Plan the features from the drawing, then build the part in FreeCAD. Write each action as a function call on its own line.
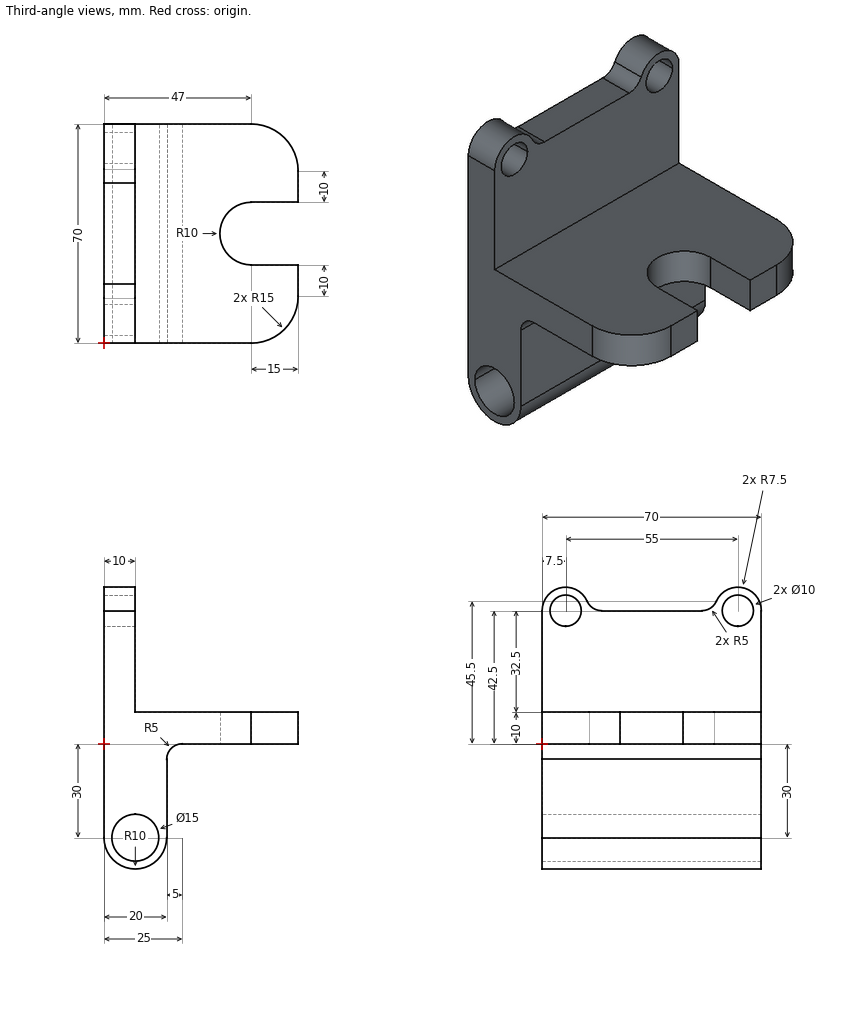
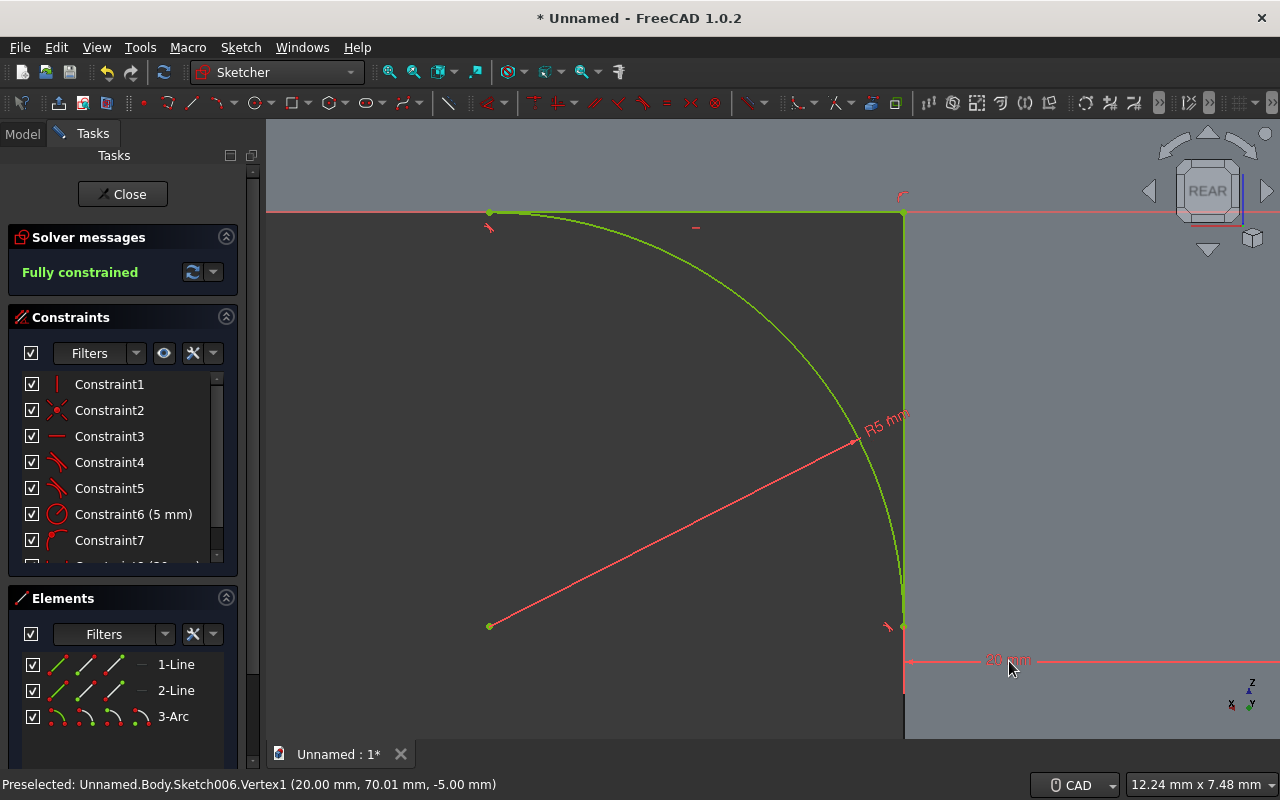
click(123, 194)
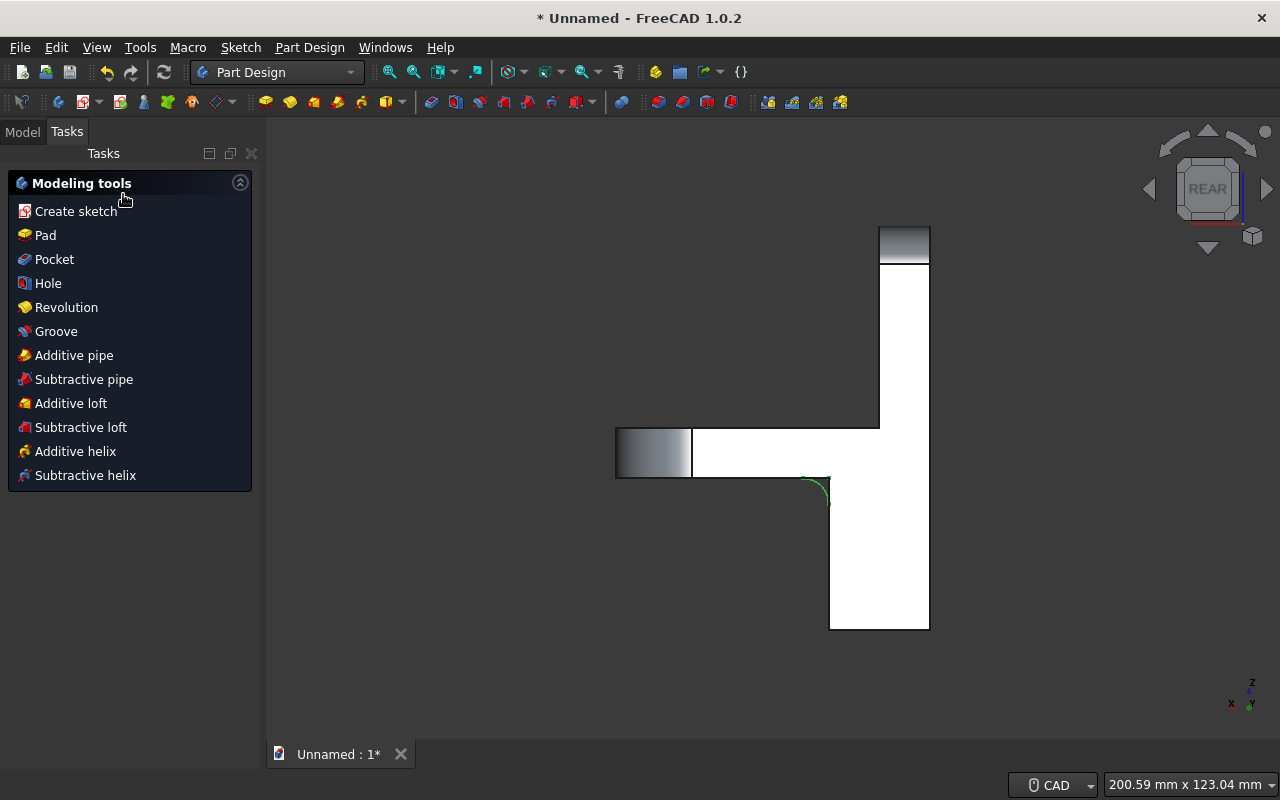
click(266, 102)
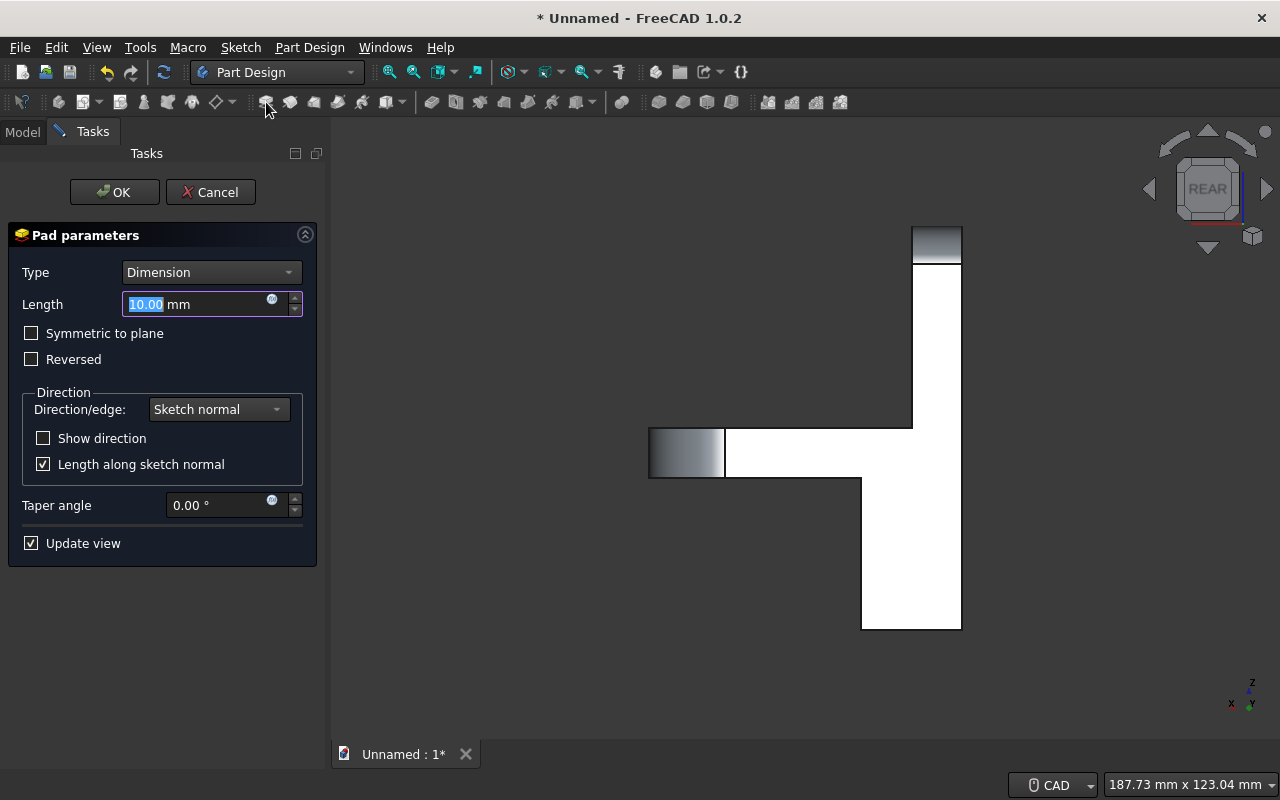
text(70)
key(Tab)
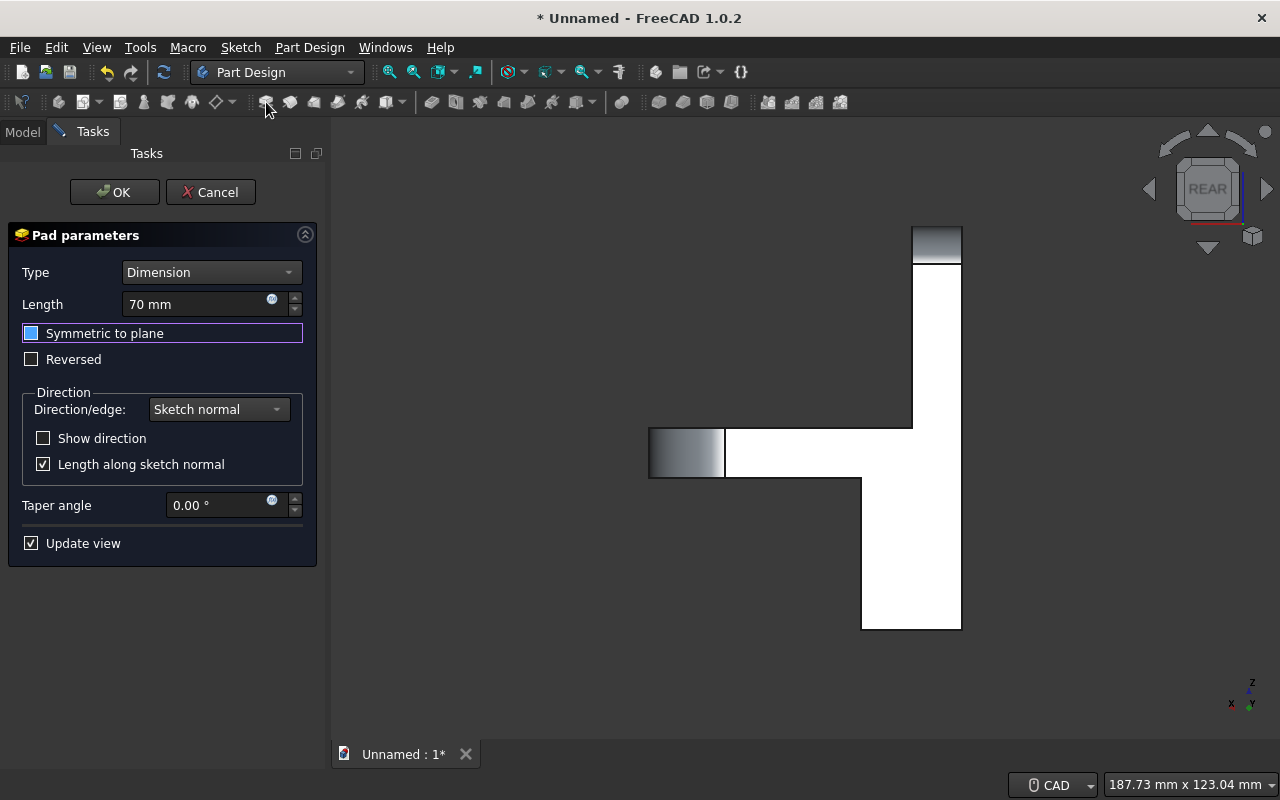
click(30, 359)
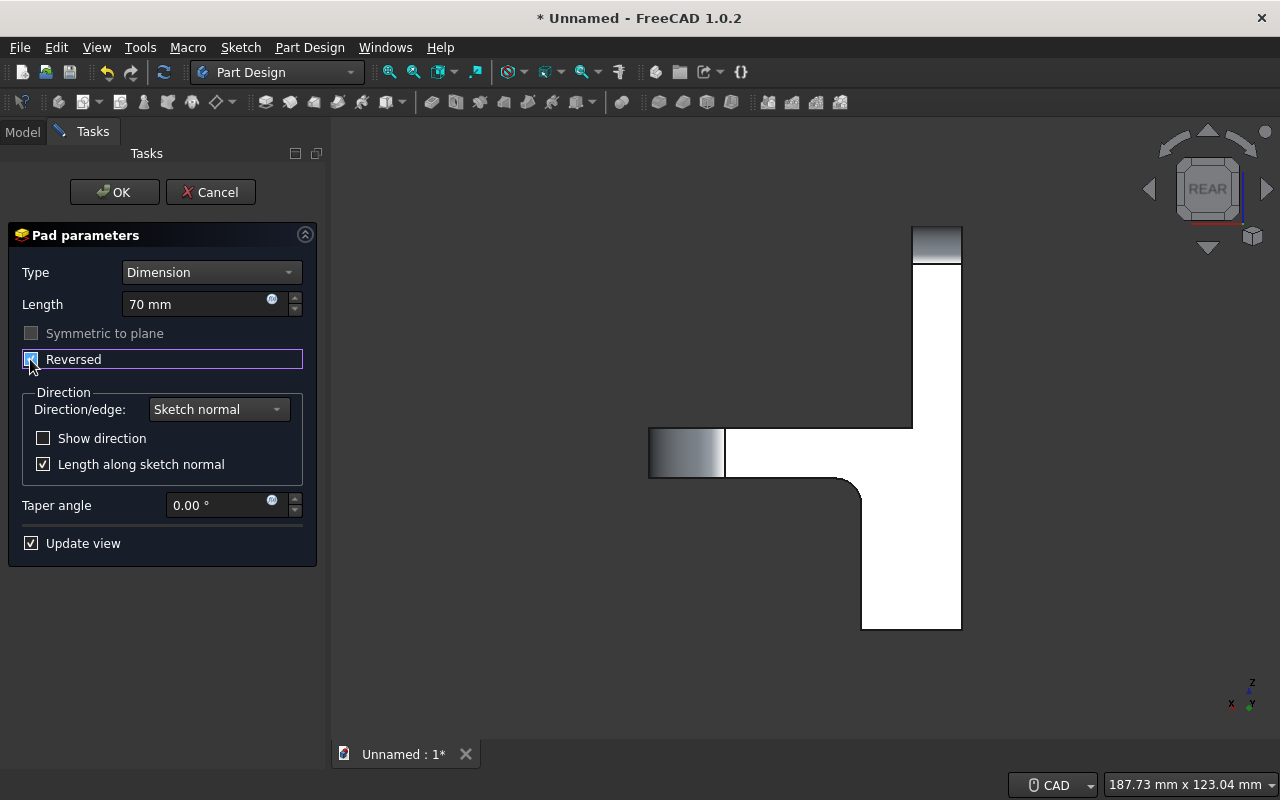
click(115, 192)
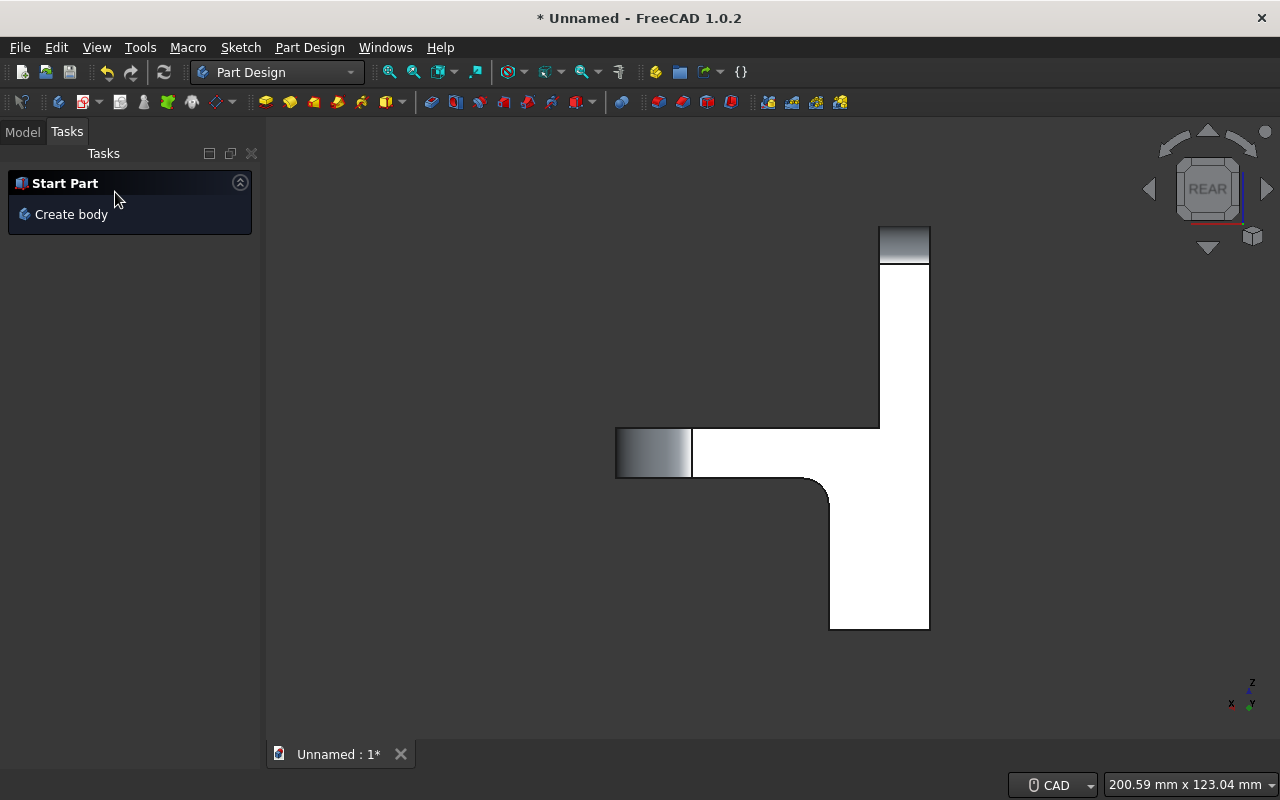
click(879, 498)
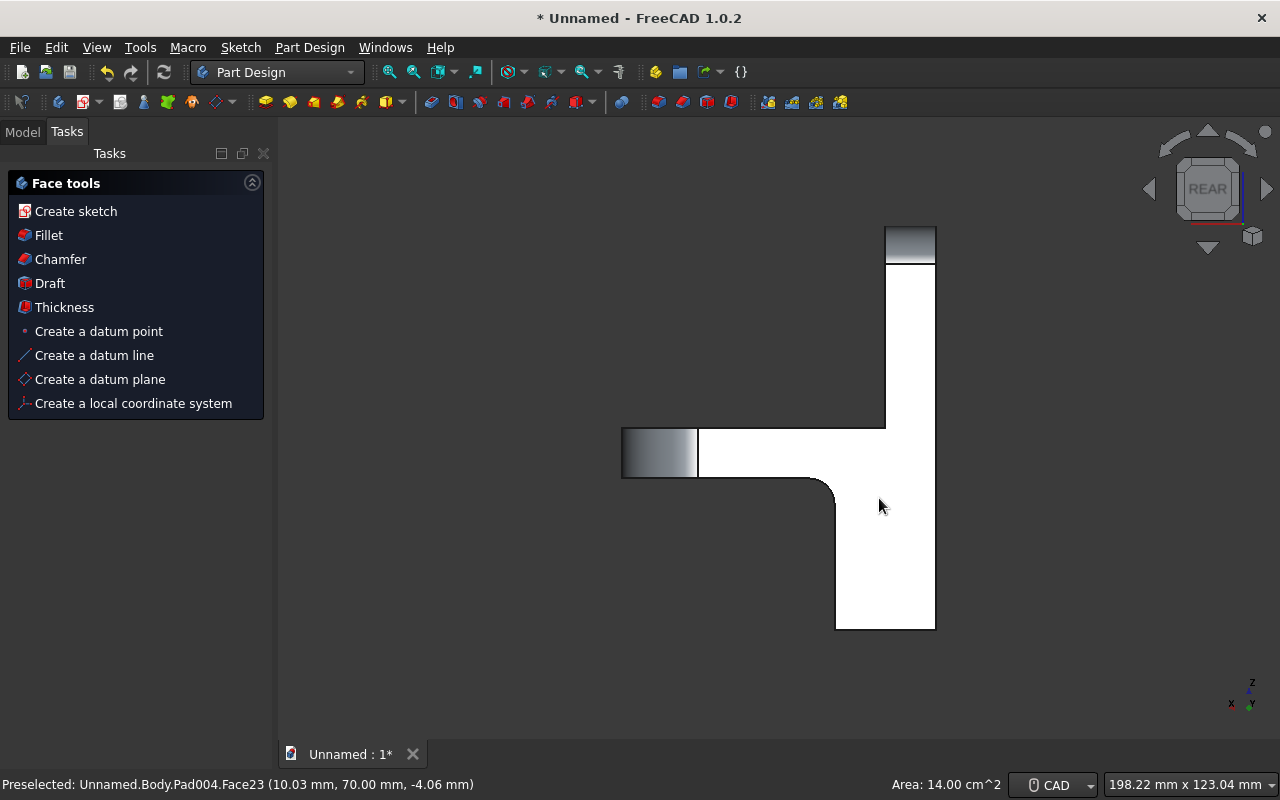
click(84, 102)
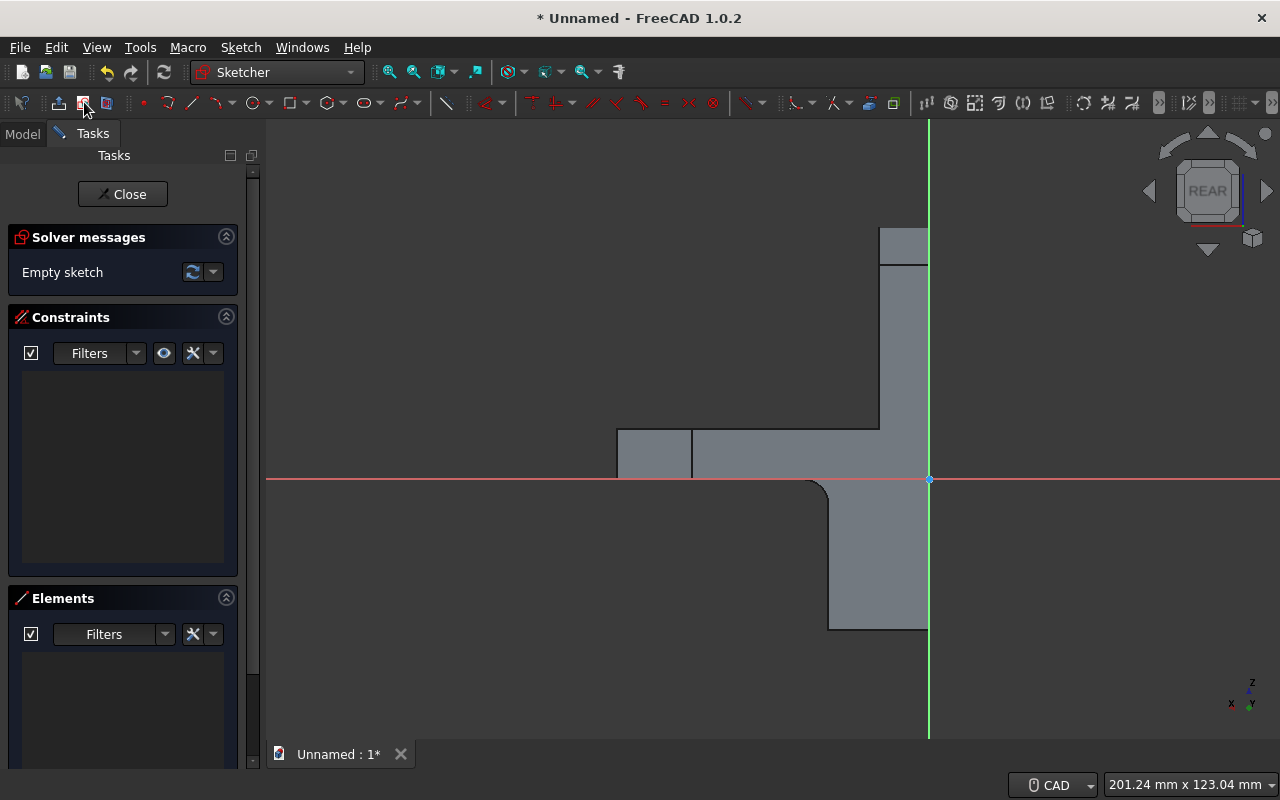
scroll(1091, 711, up, 3)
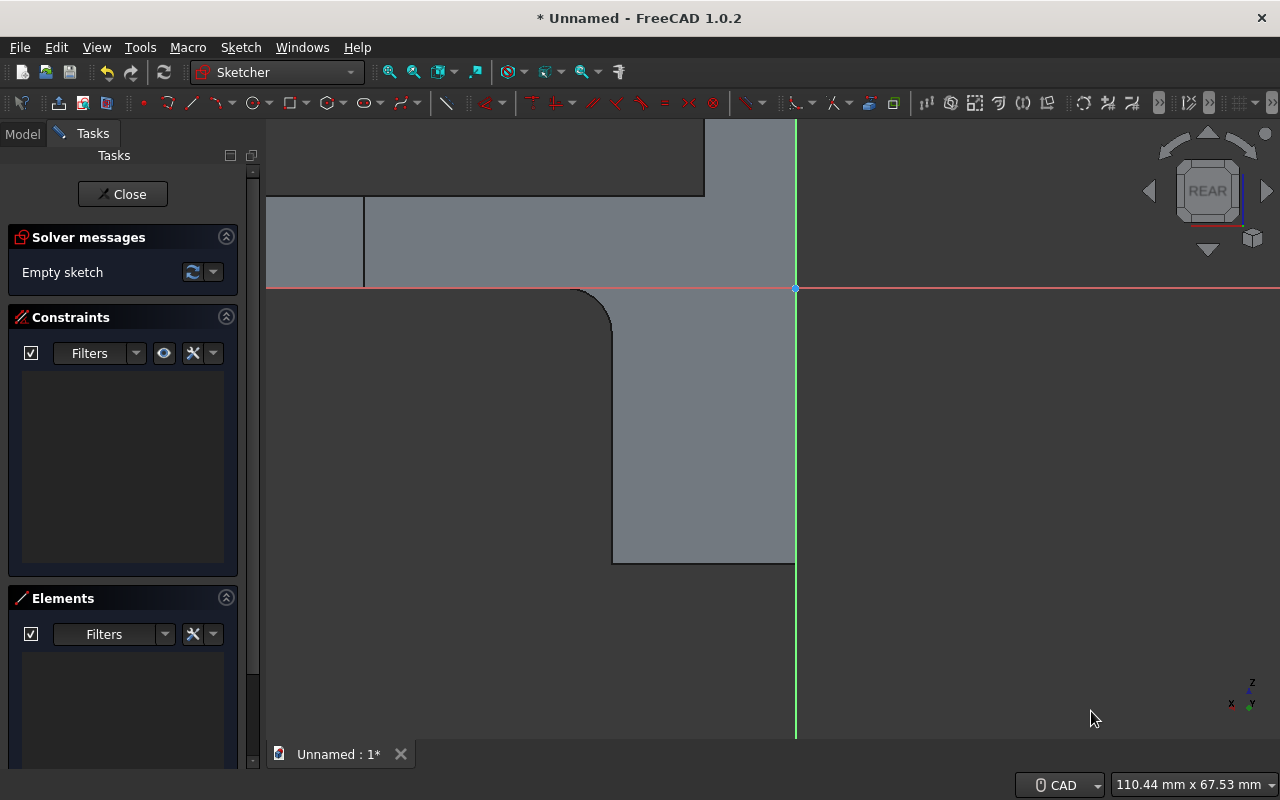
click(192, 104)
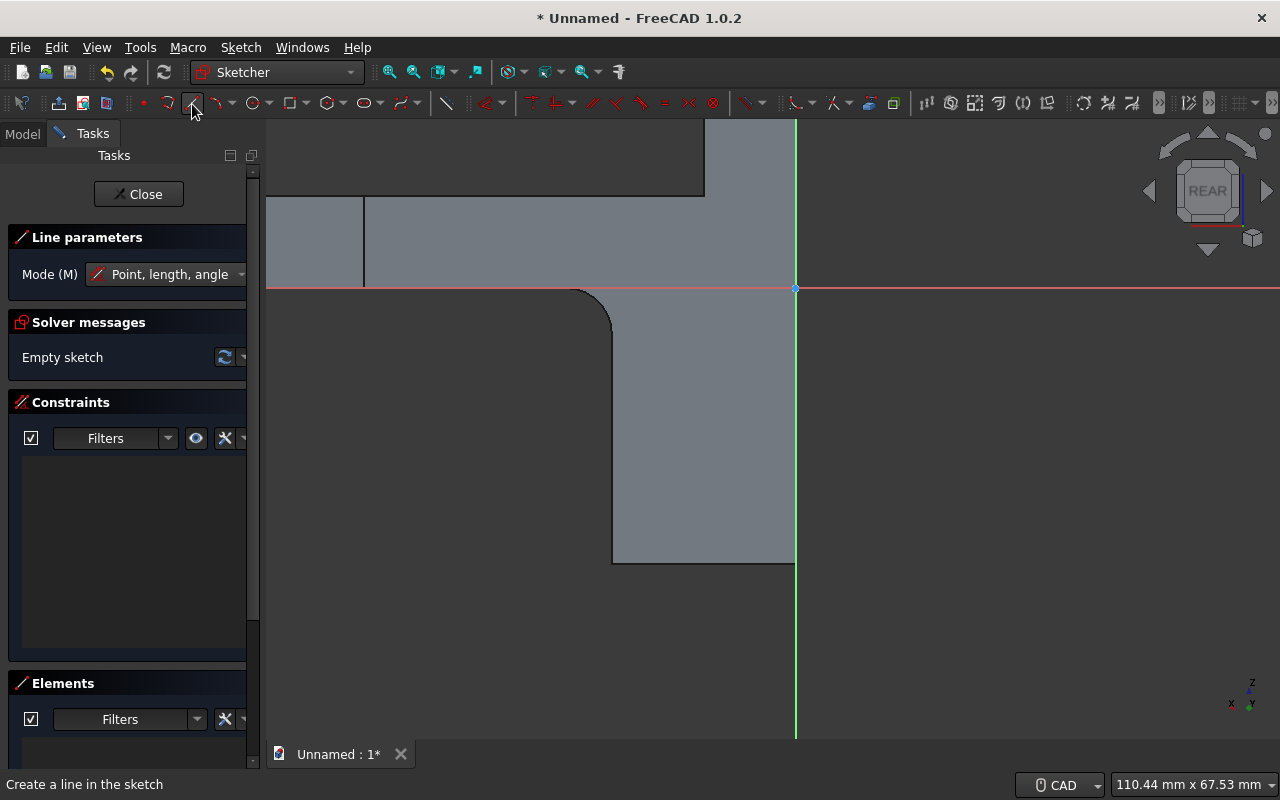
click(796, 564)
click(612, 564)